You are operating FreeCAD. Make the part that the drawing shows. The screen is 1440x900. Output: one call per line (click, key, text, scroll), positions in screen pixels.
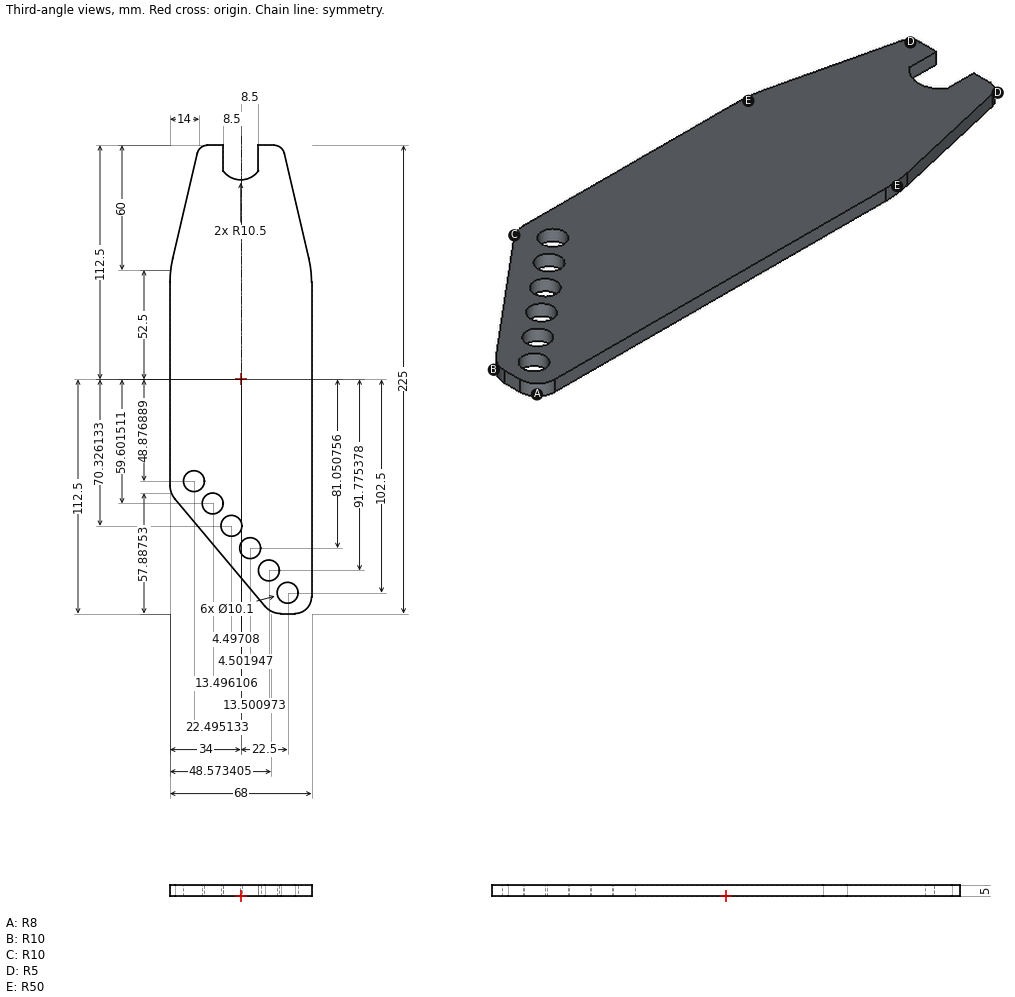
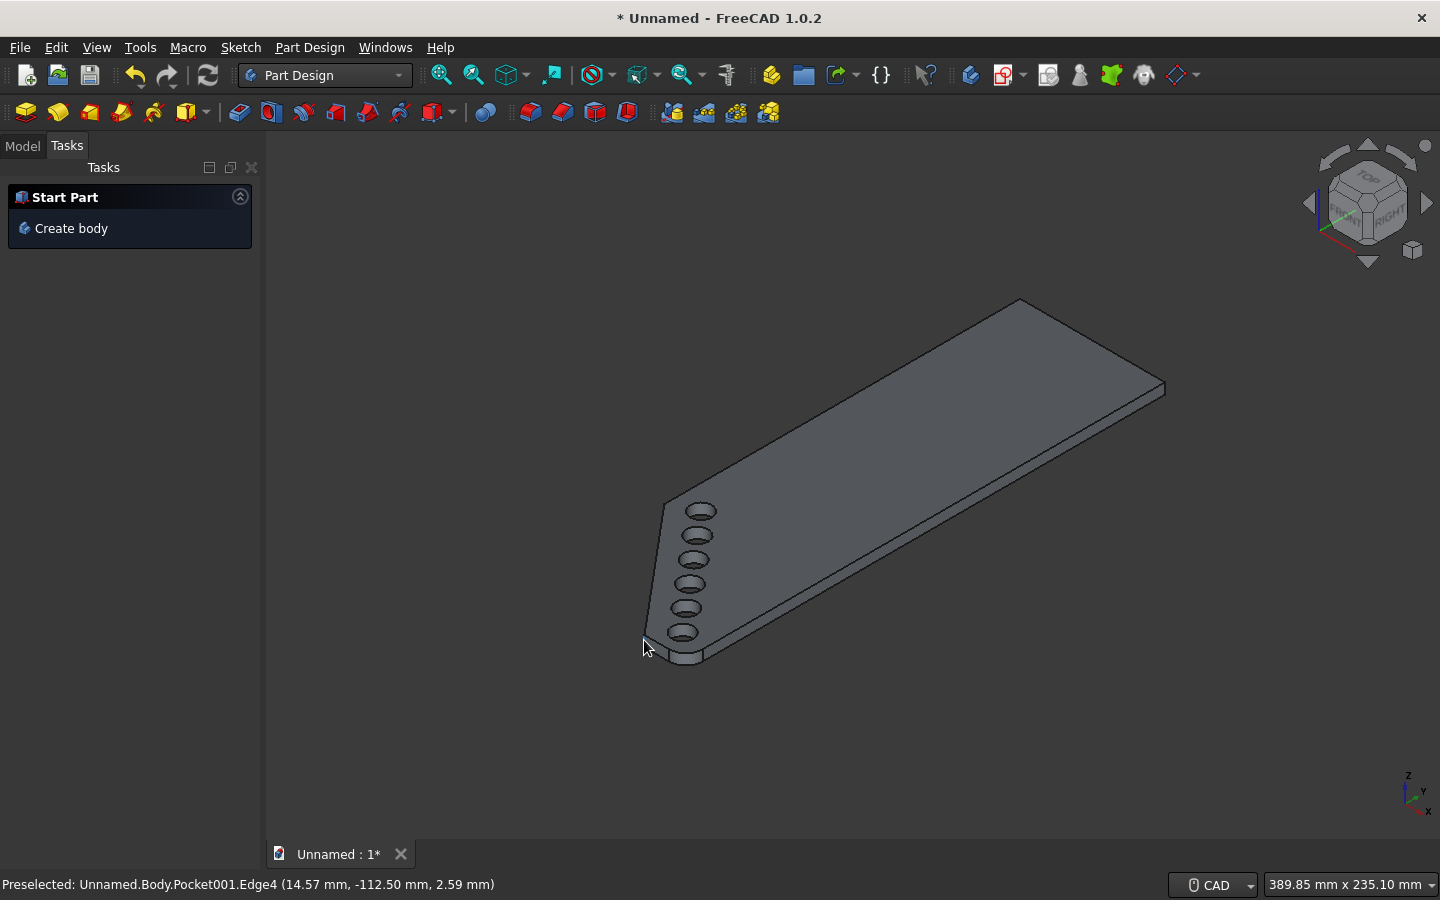
key(2)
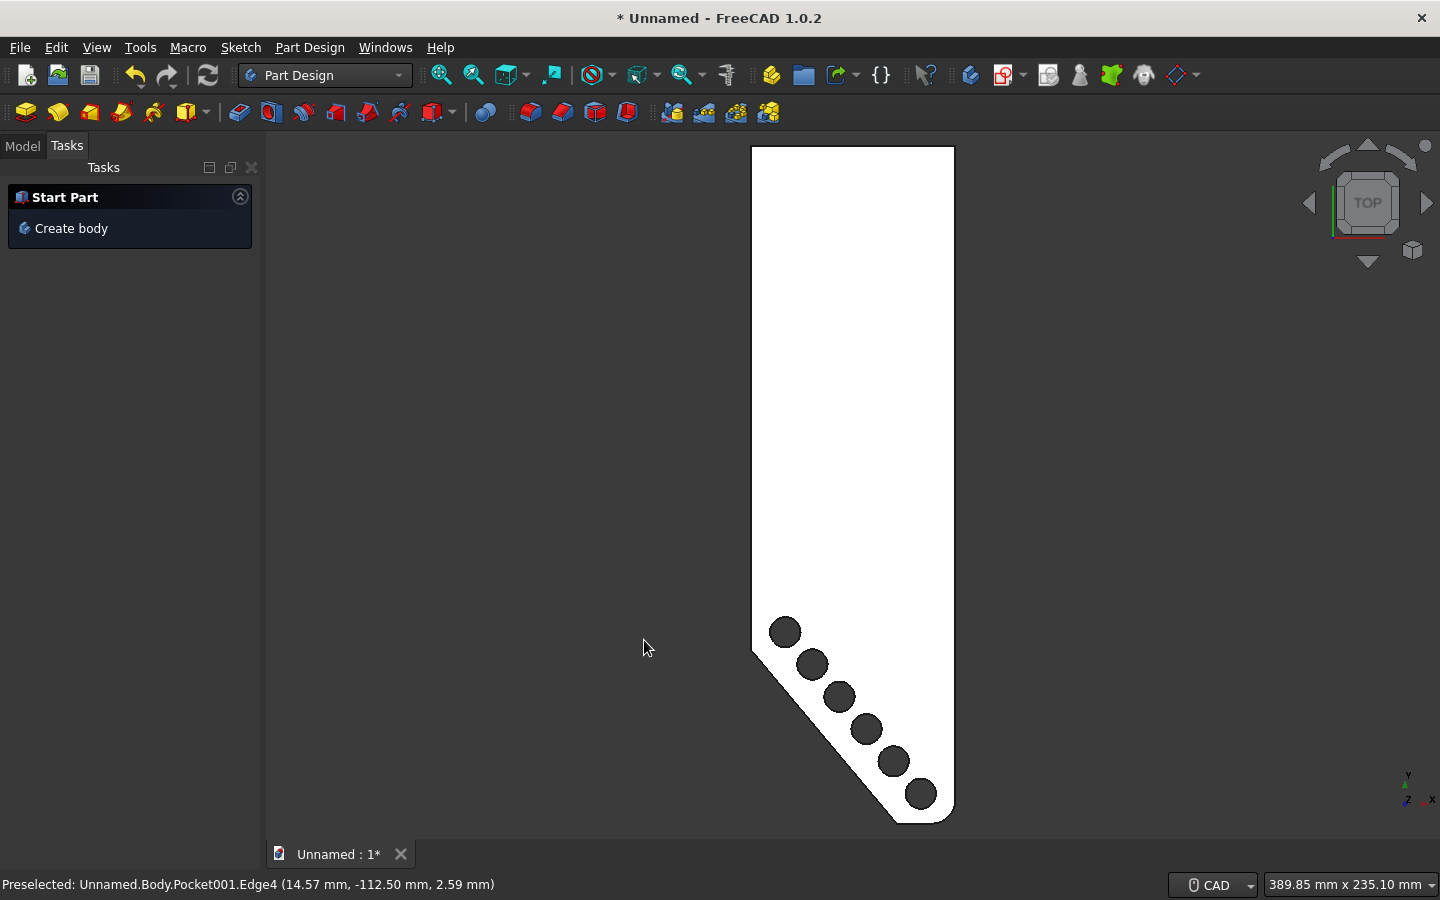
key(1)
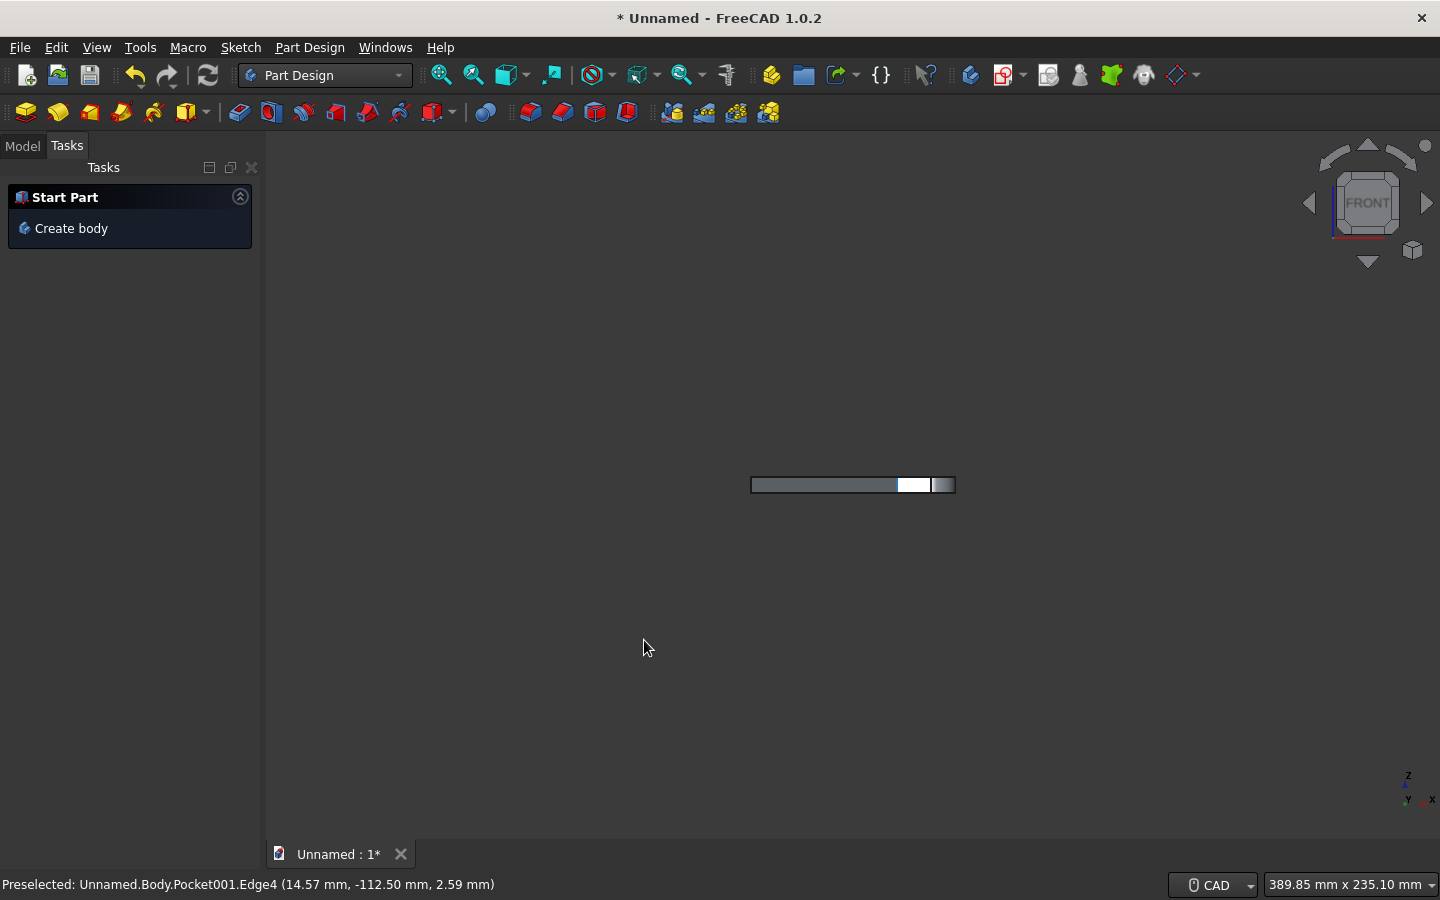
key(v)
key(f)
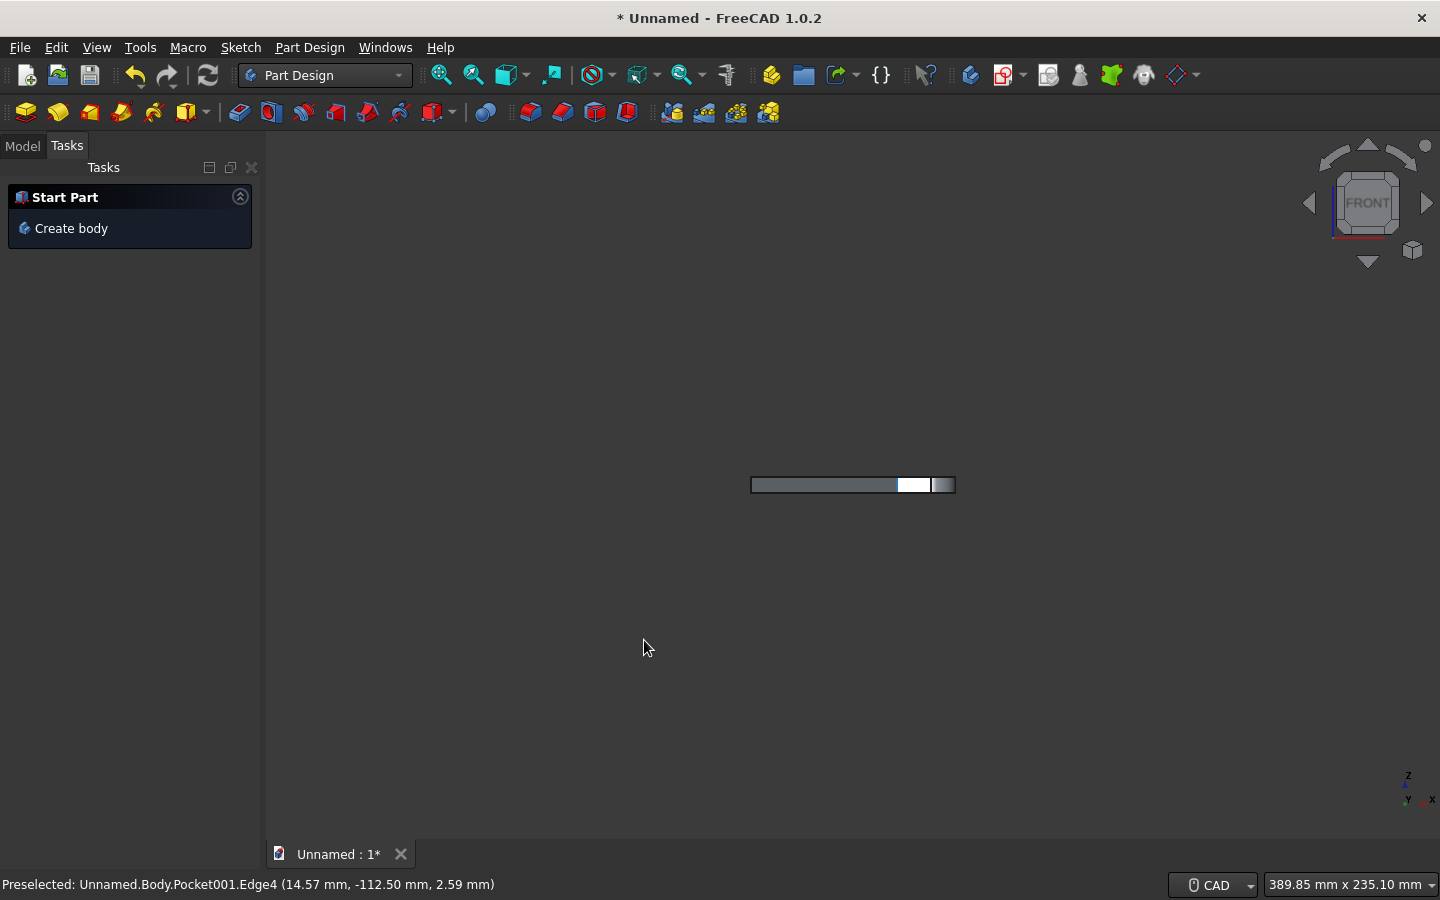
click(897, 484)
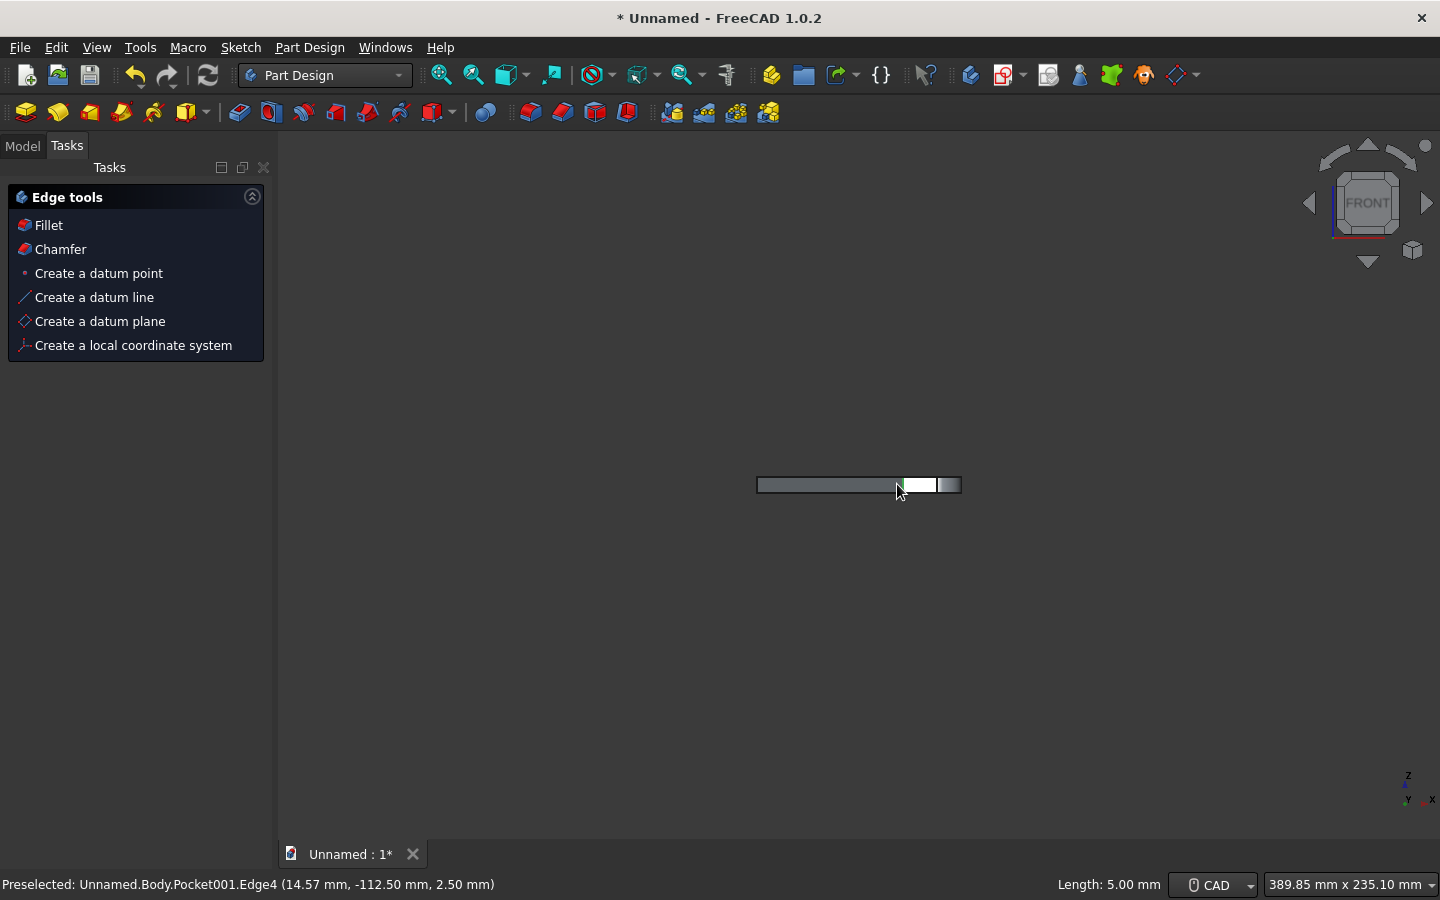
click(532, 112)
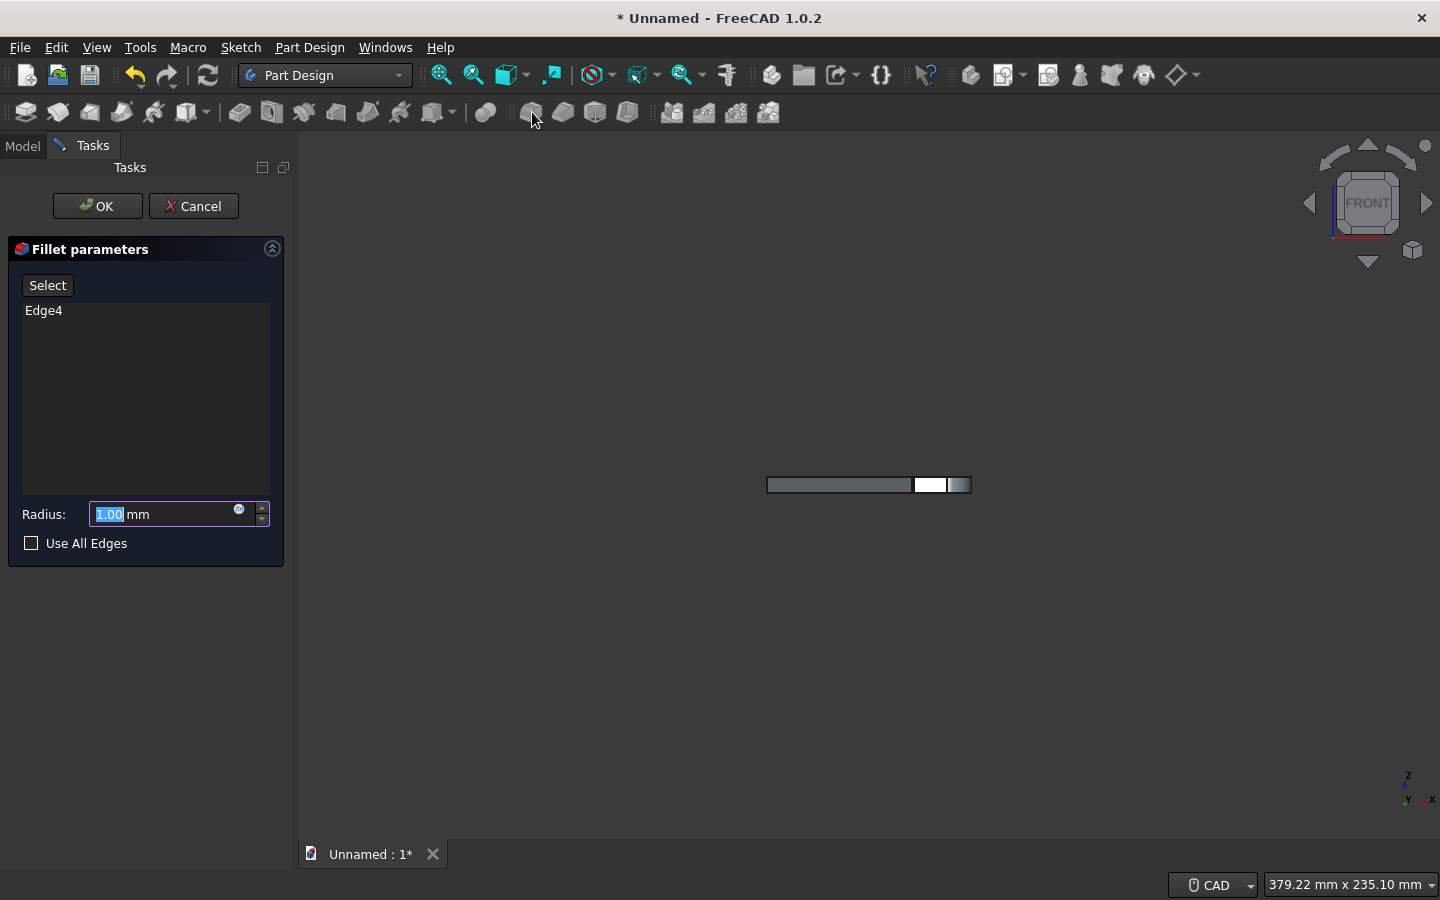
text(10)
key(Tab)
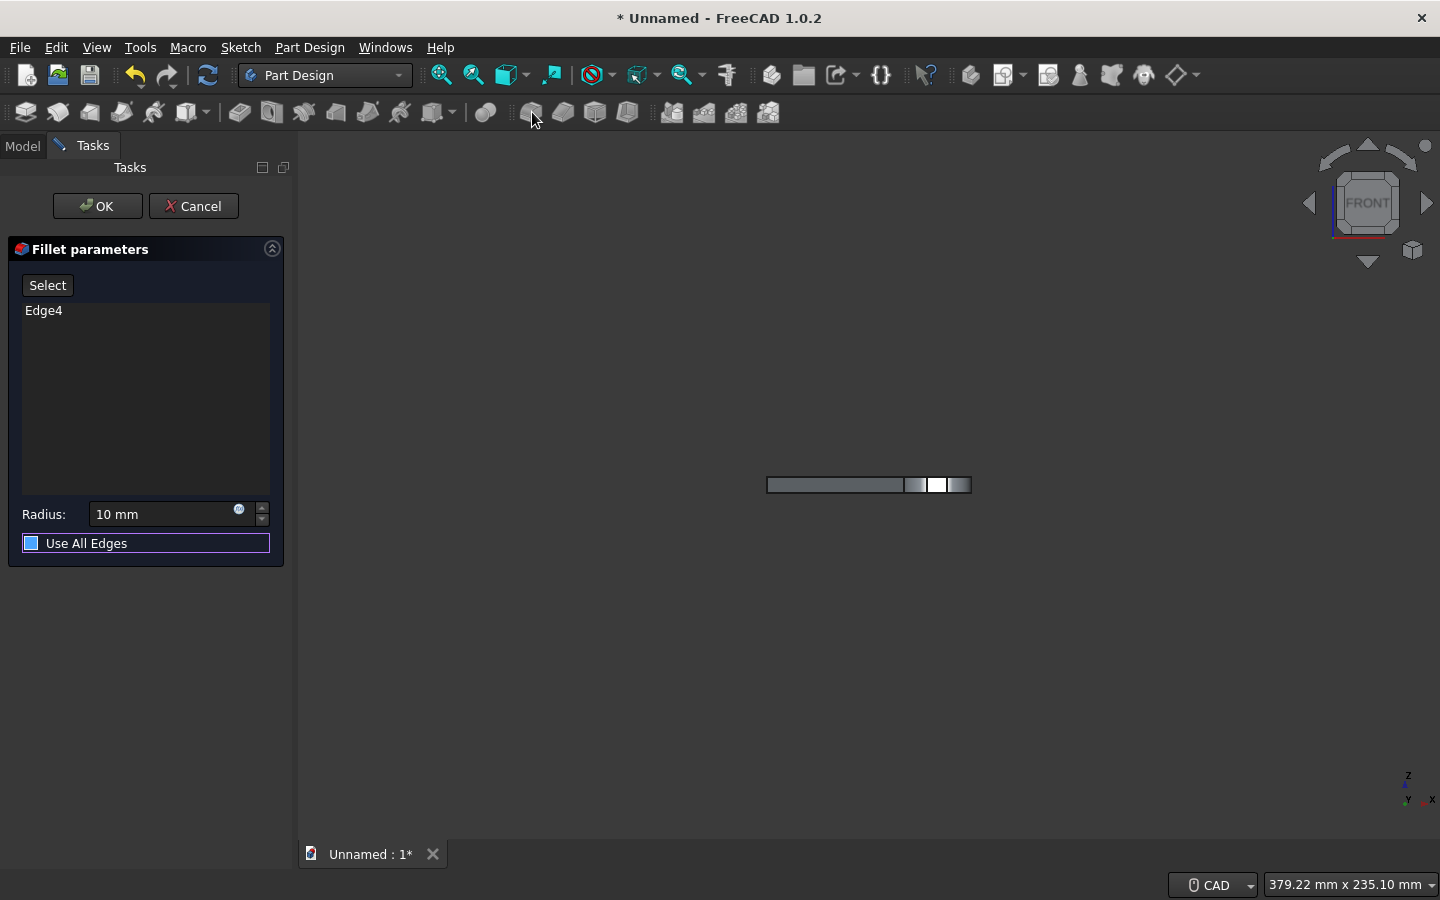
click(98, 206)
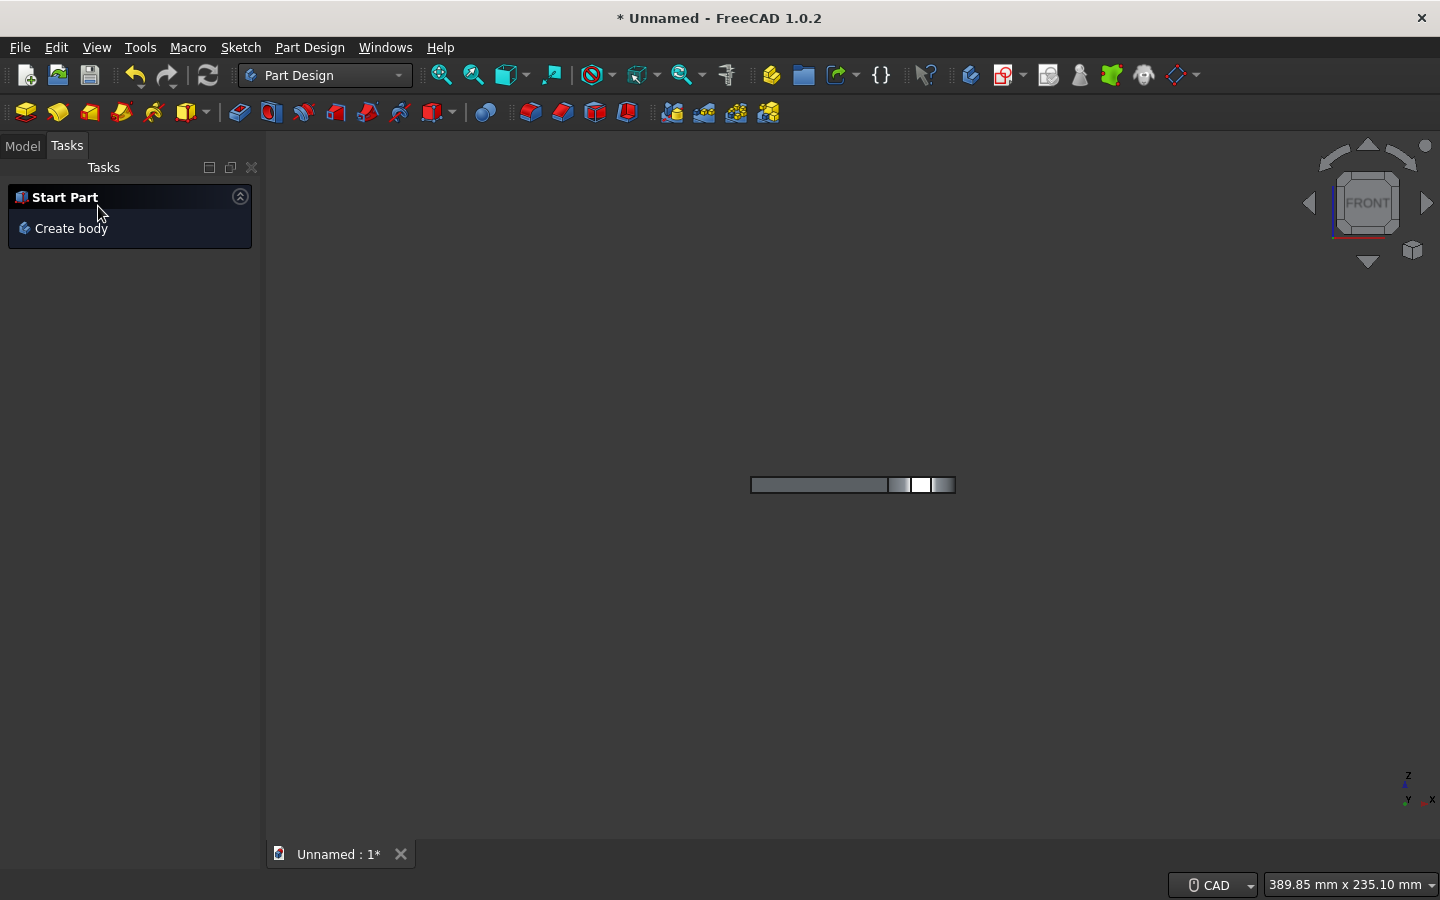
click(442, 76)